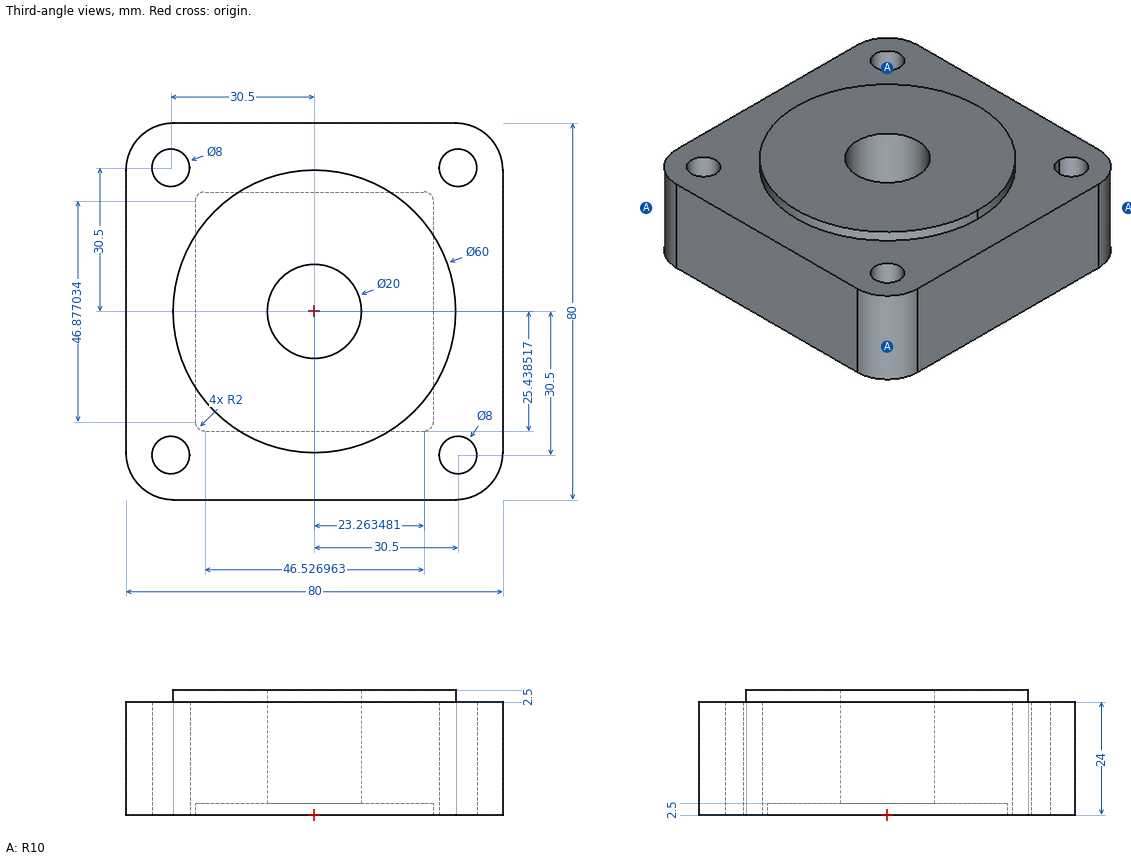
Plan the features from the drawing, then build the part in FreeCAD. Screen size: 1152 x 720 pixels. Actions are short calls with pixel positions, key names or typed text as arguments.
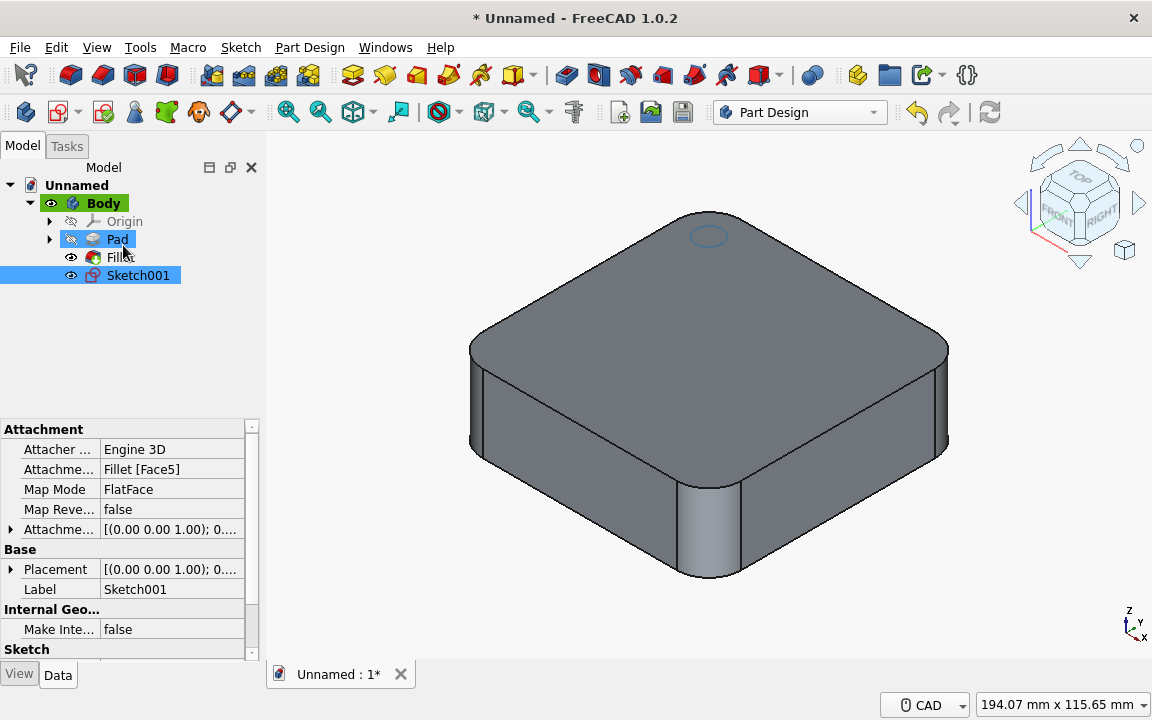
click(568, 76)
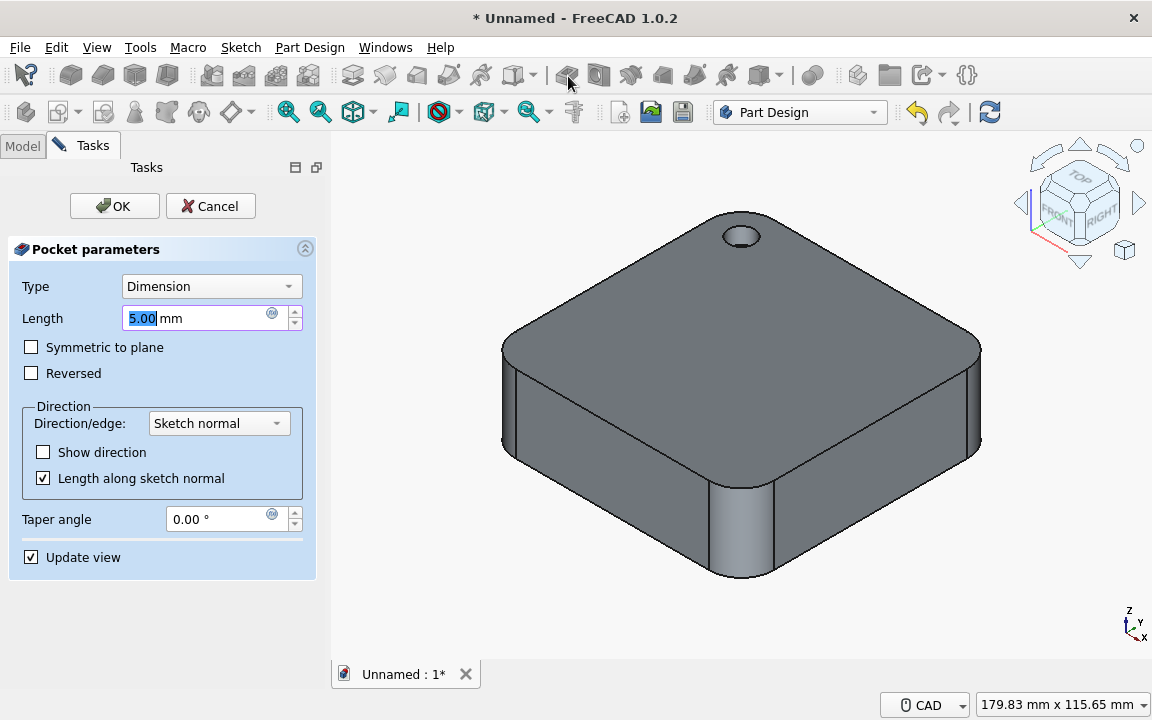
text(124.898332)
key(Tab)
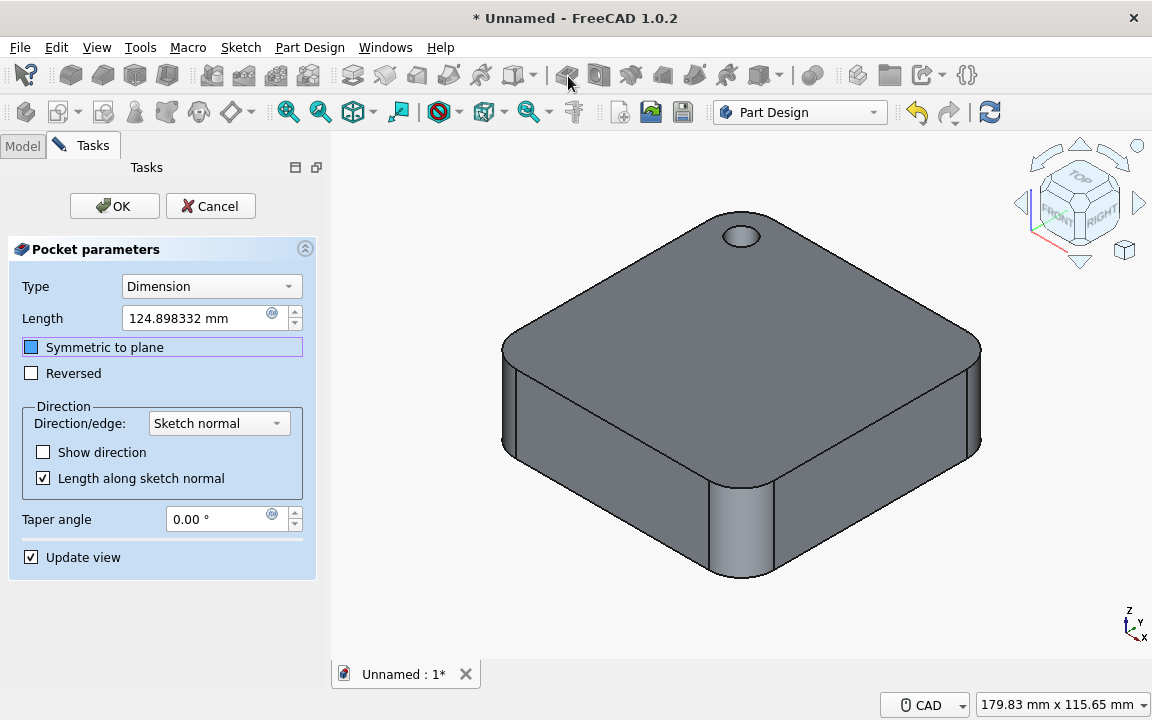
click(30, 347)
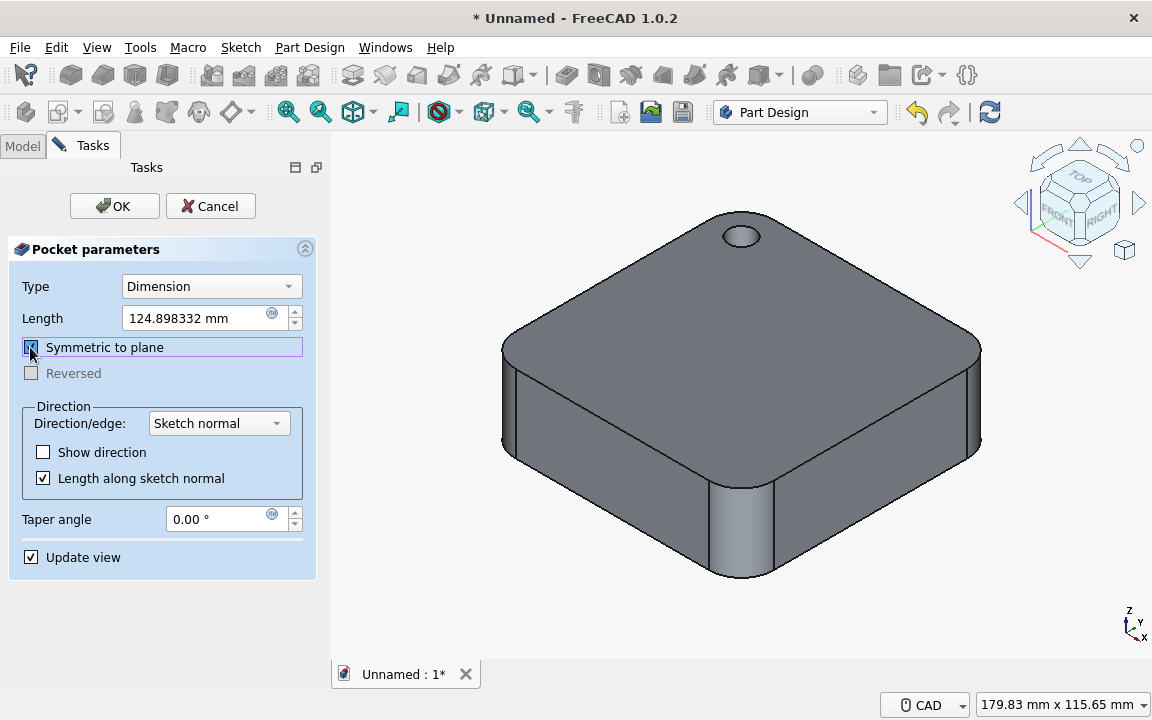
click(115, 206)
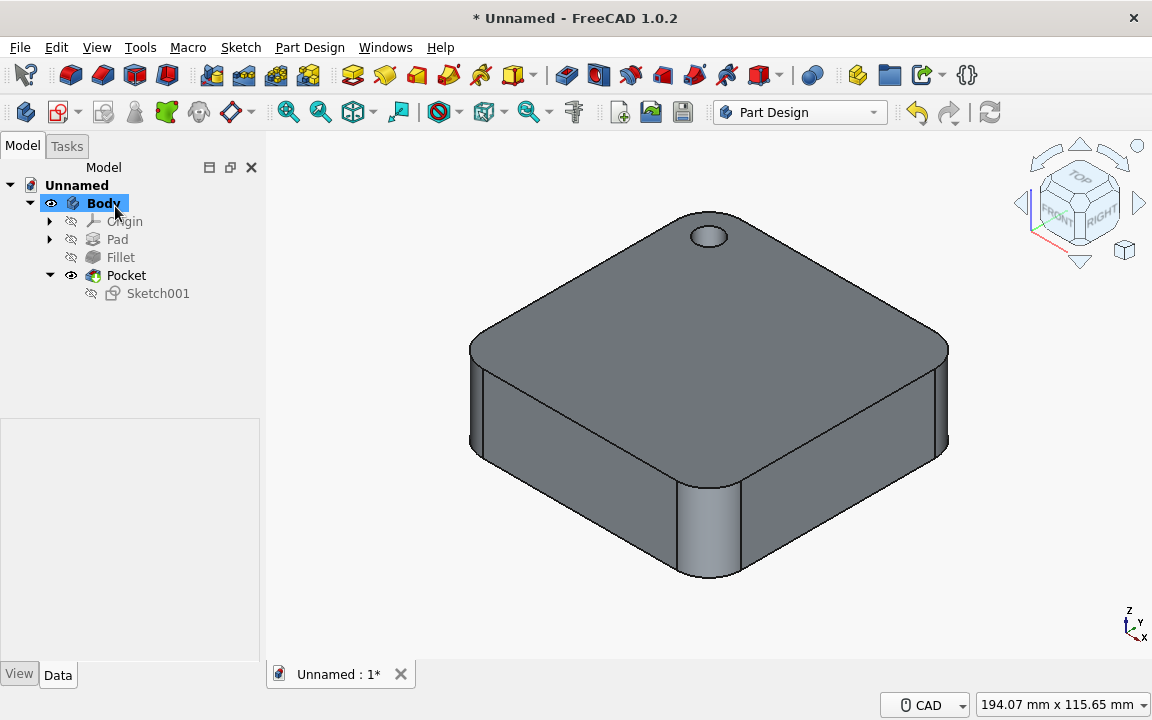
click(116, 275)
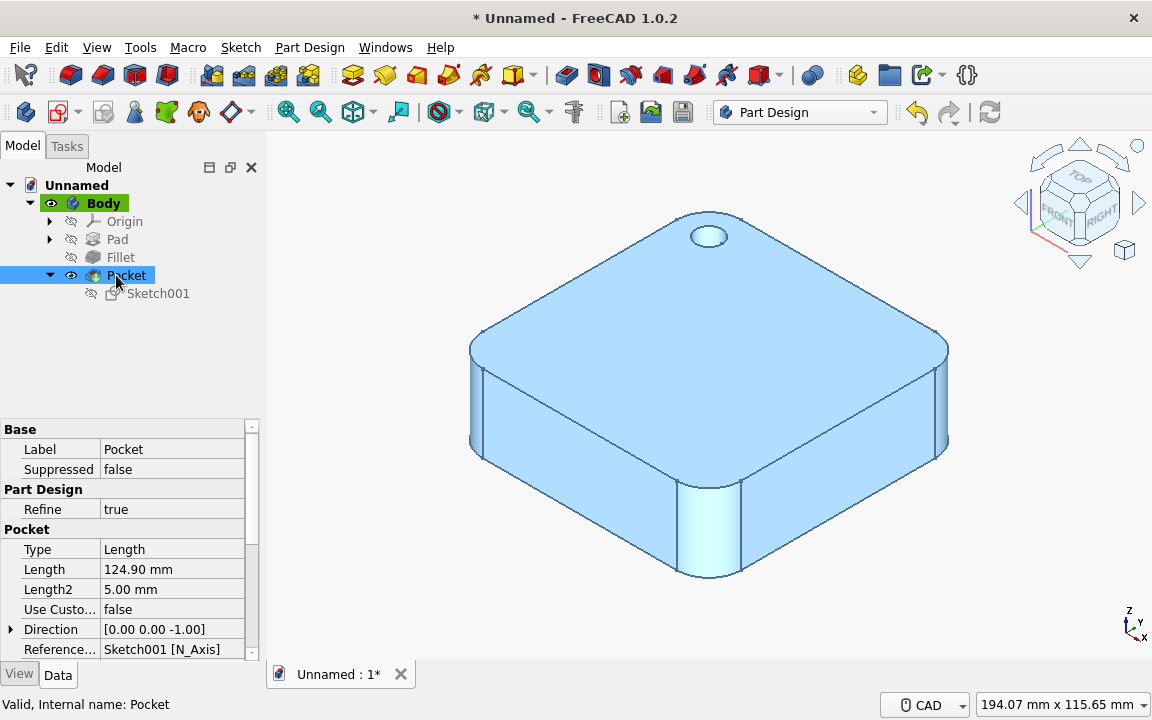
click(212, 76)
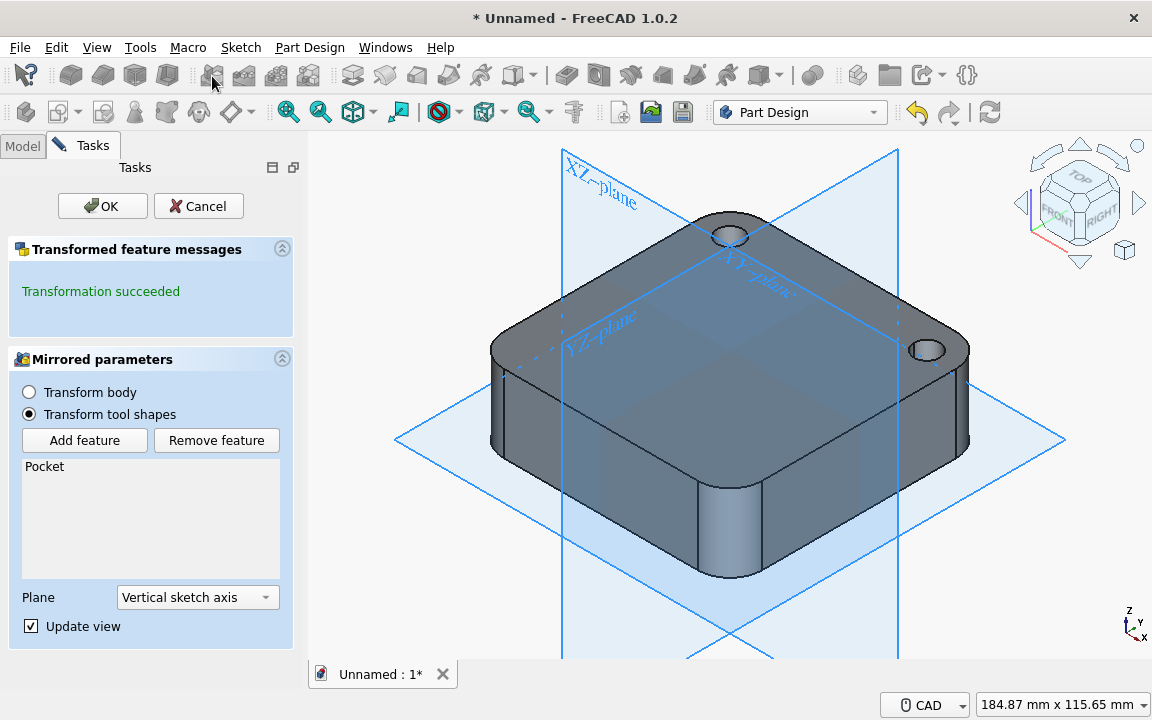
click(198, 598)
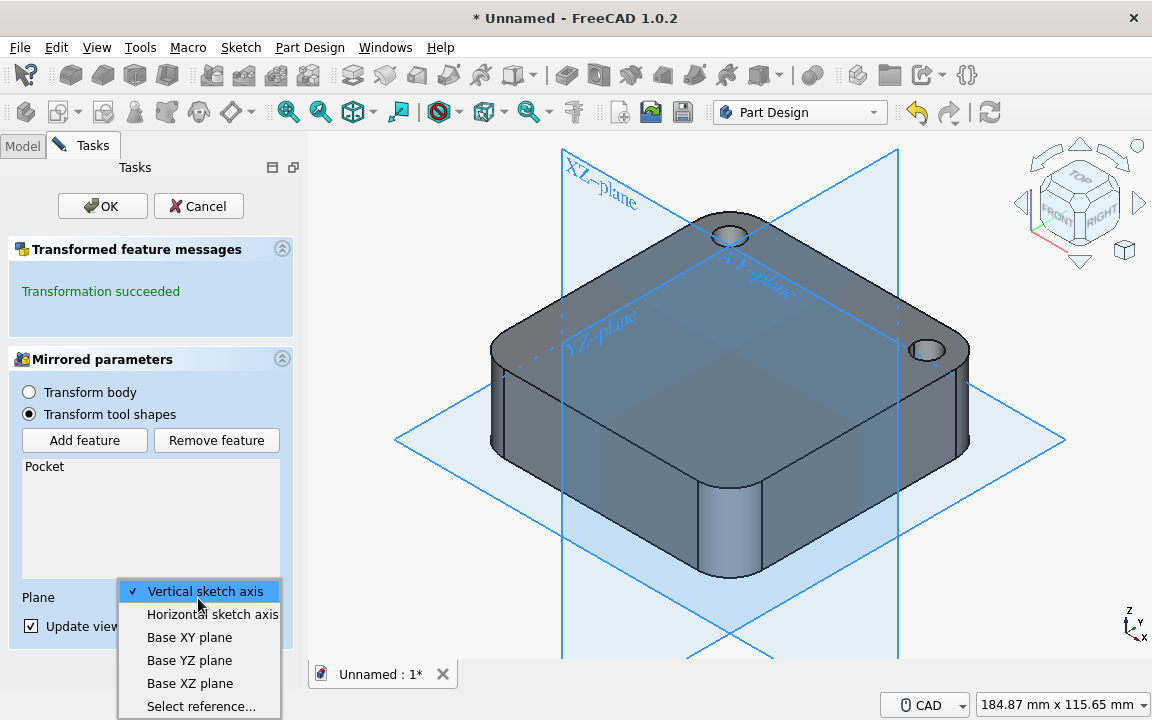
click(198, 684)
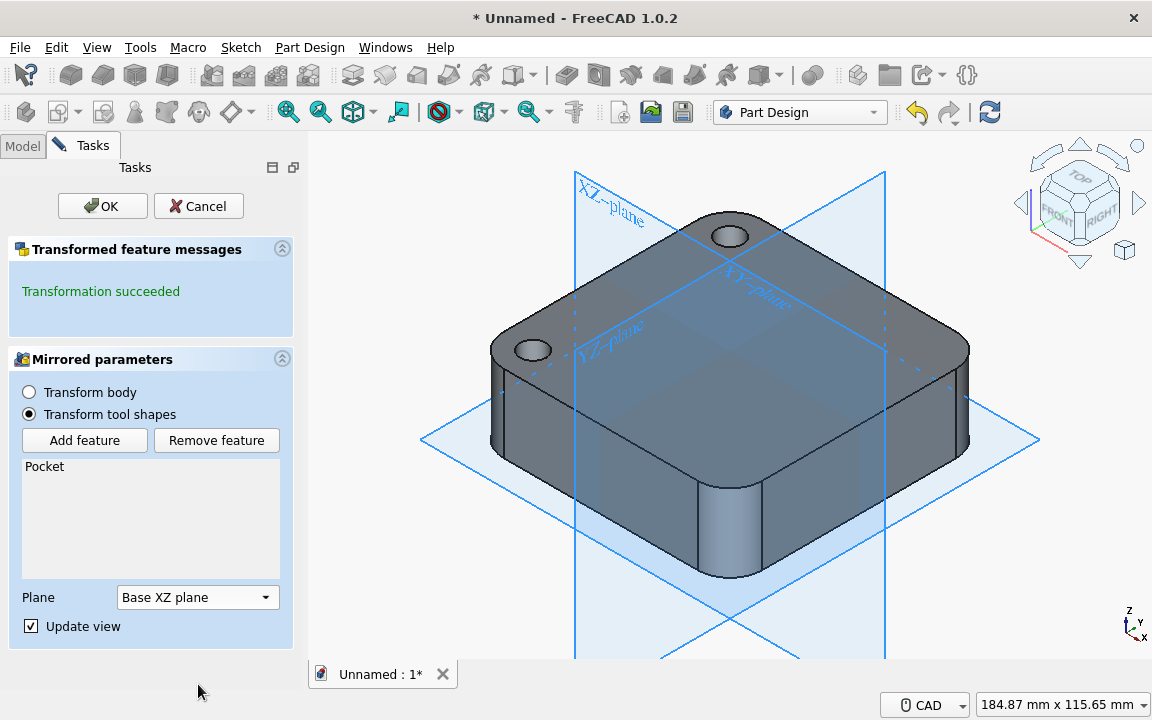
click(103, 206)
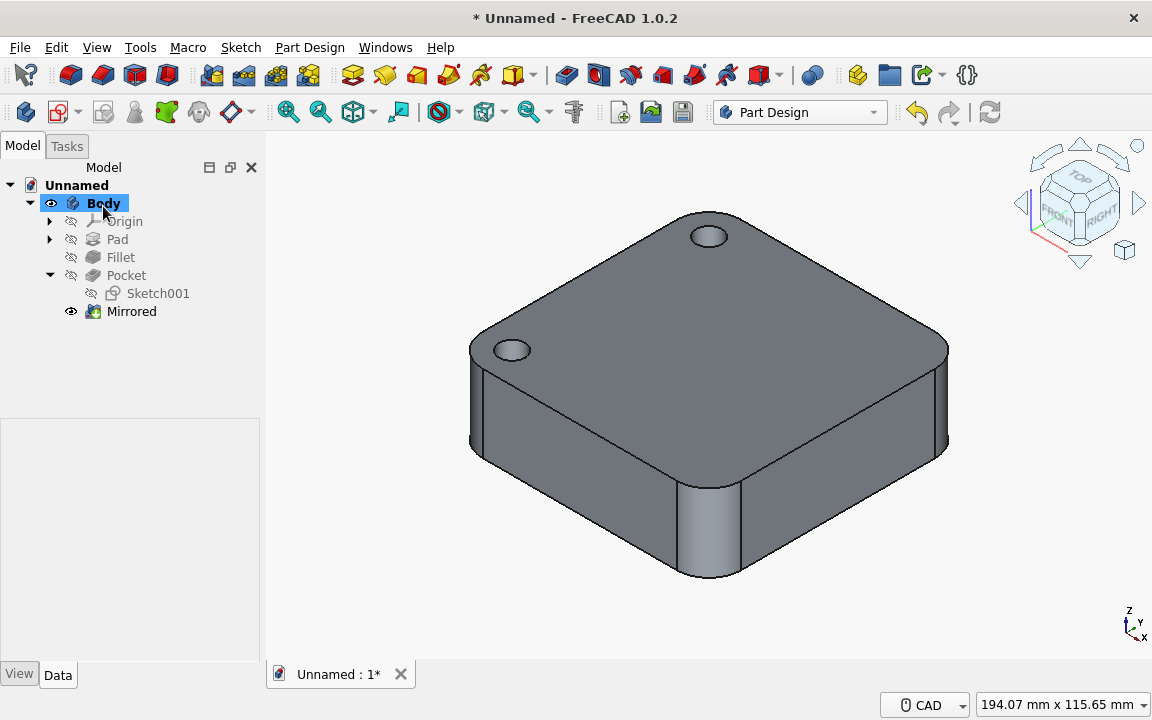
click(116, 275)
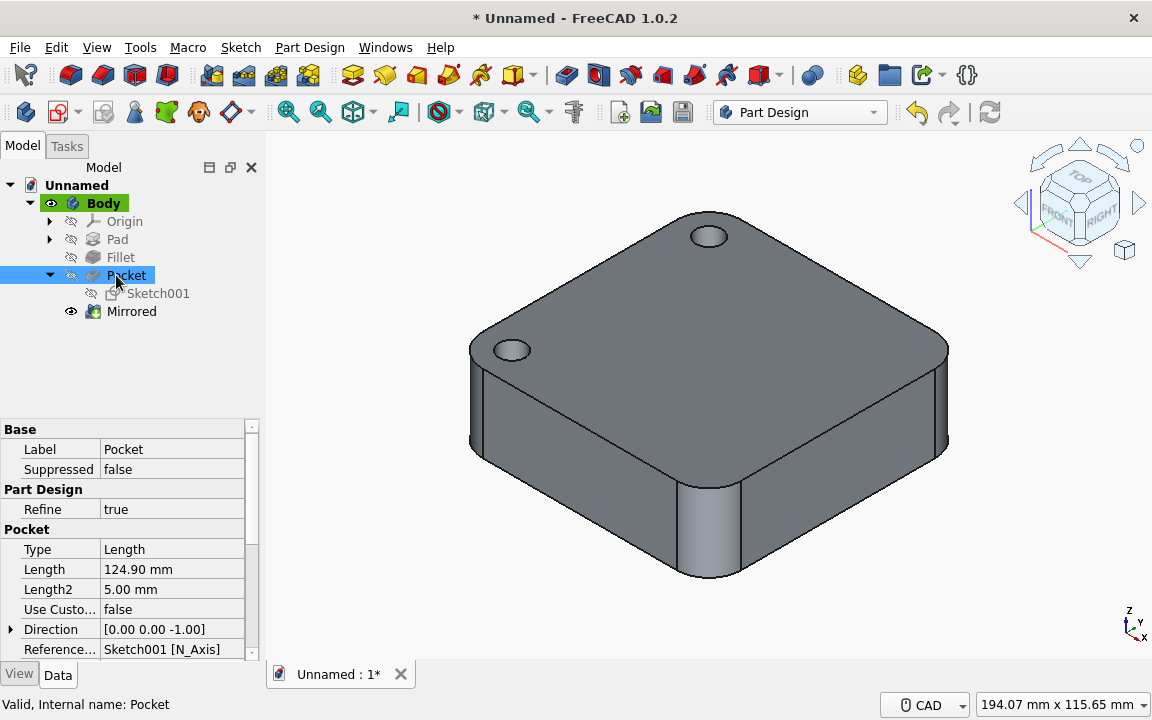
click(212, 76)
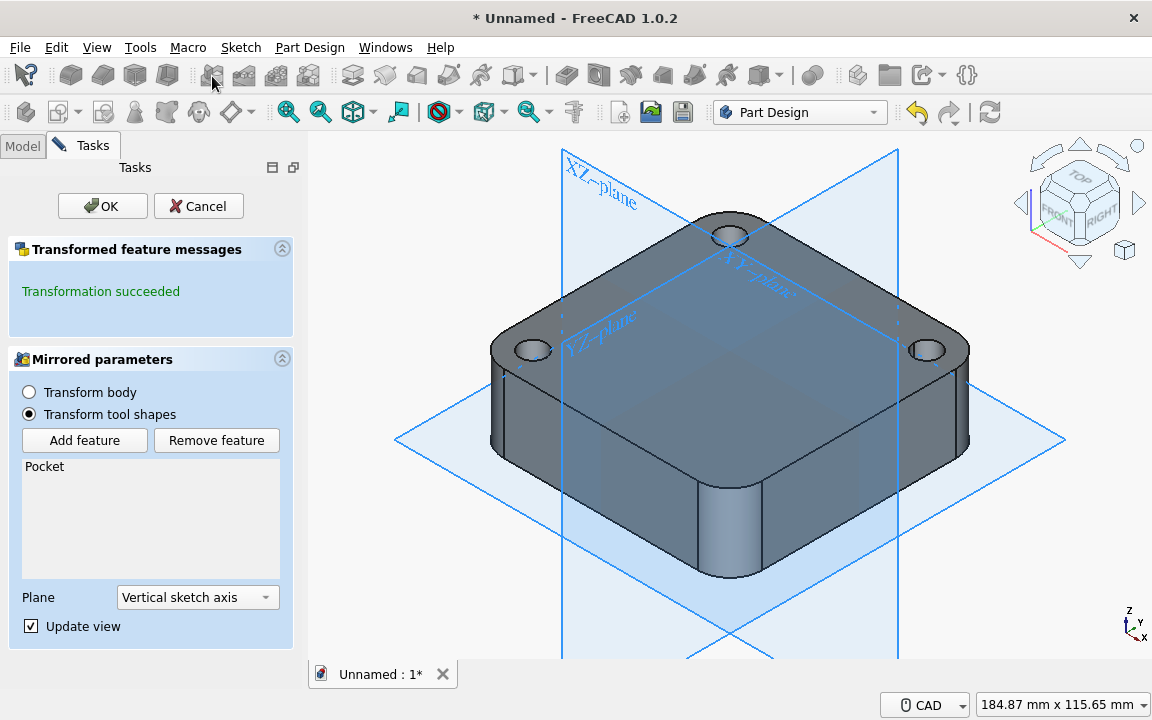
click(198, 598)